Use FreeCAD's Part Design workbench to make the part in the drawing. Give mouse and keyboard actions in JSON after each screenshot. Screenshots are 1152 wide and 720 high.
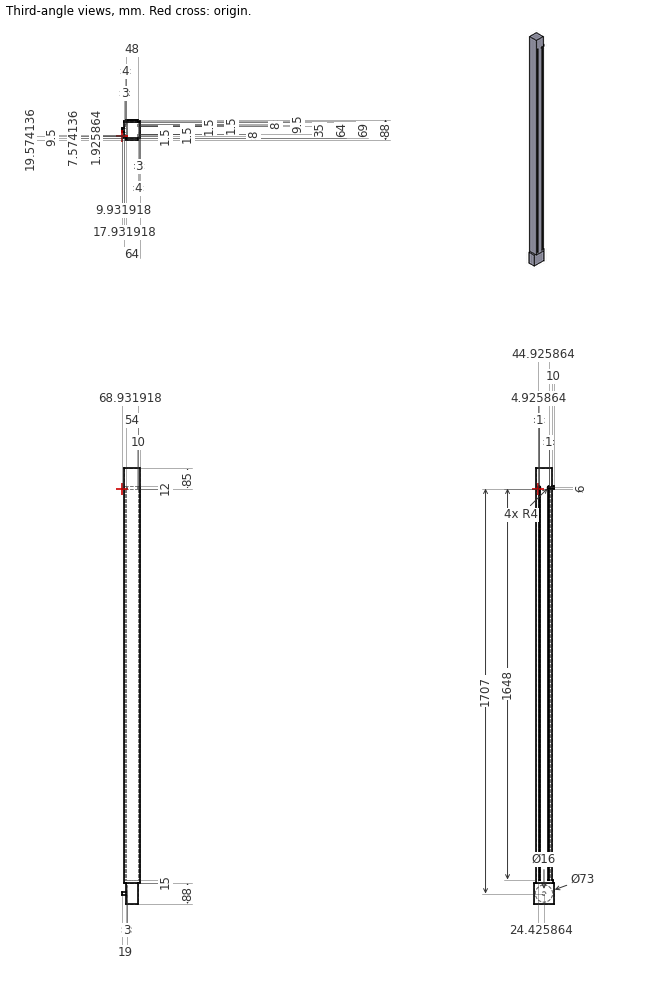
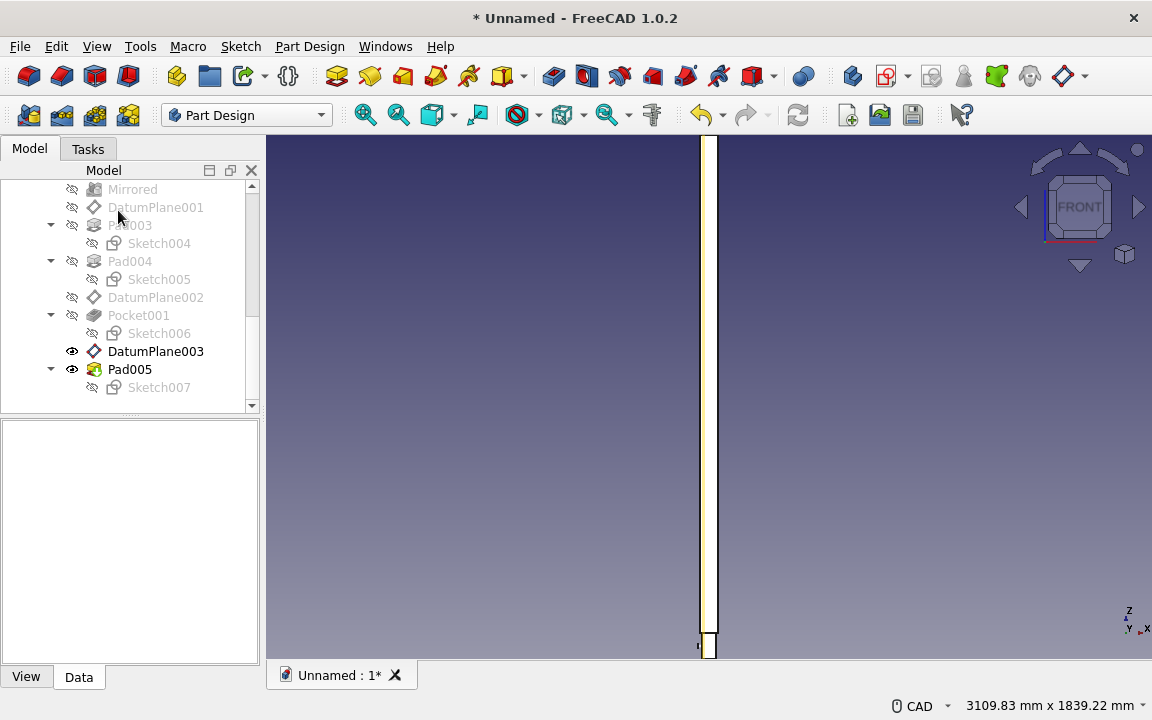
{"action": "left_click", "coordinate": [117, 351]}
{"action": "key", "text": "space"}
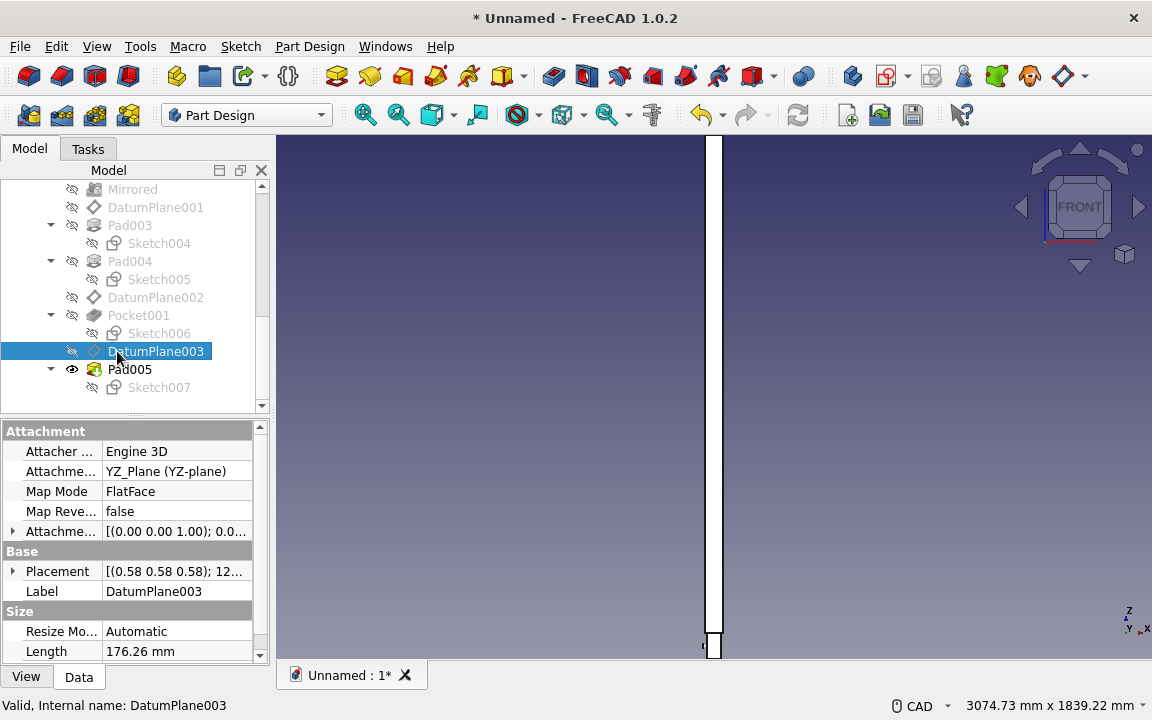
{"action": "key", "text": "0"}